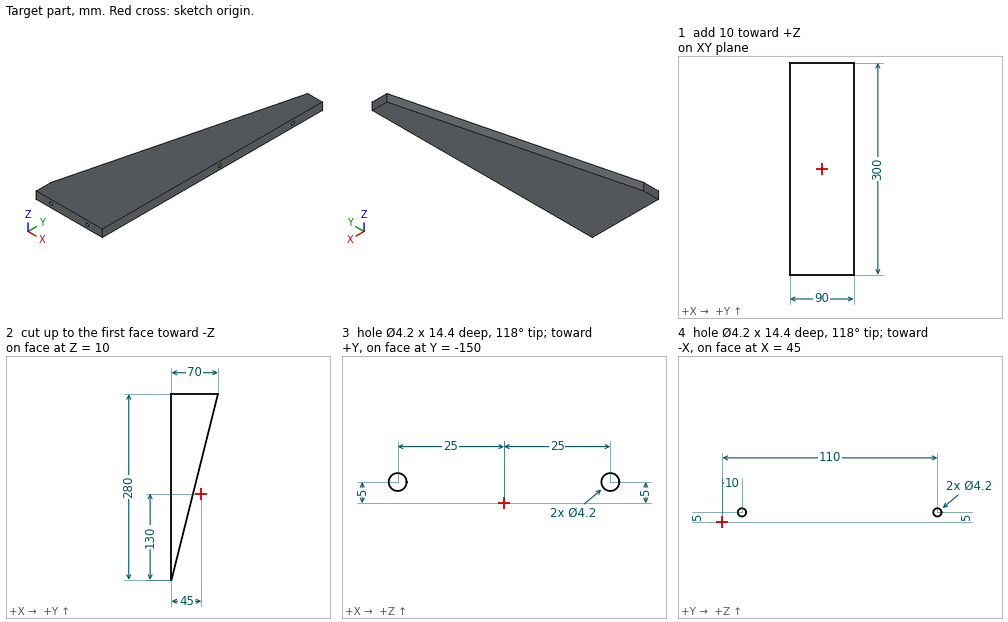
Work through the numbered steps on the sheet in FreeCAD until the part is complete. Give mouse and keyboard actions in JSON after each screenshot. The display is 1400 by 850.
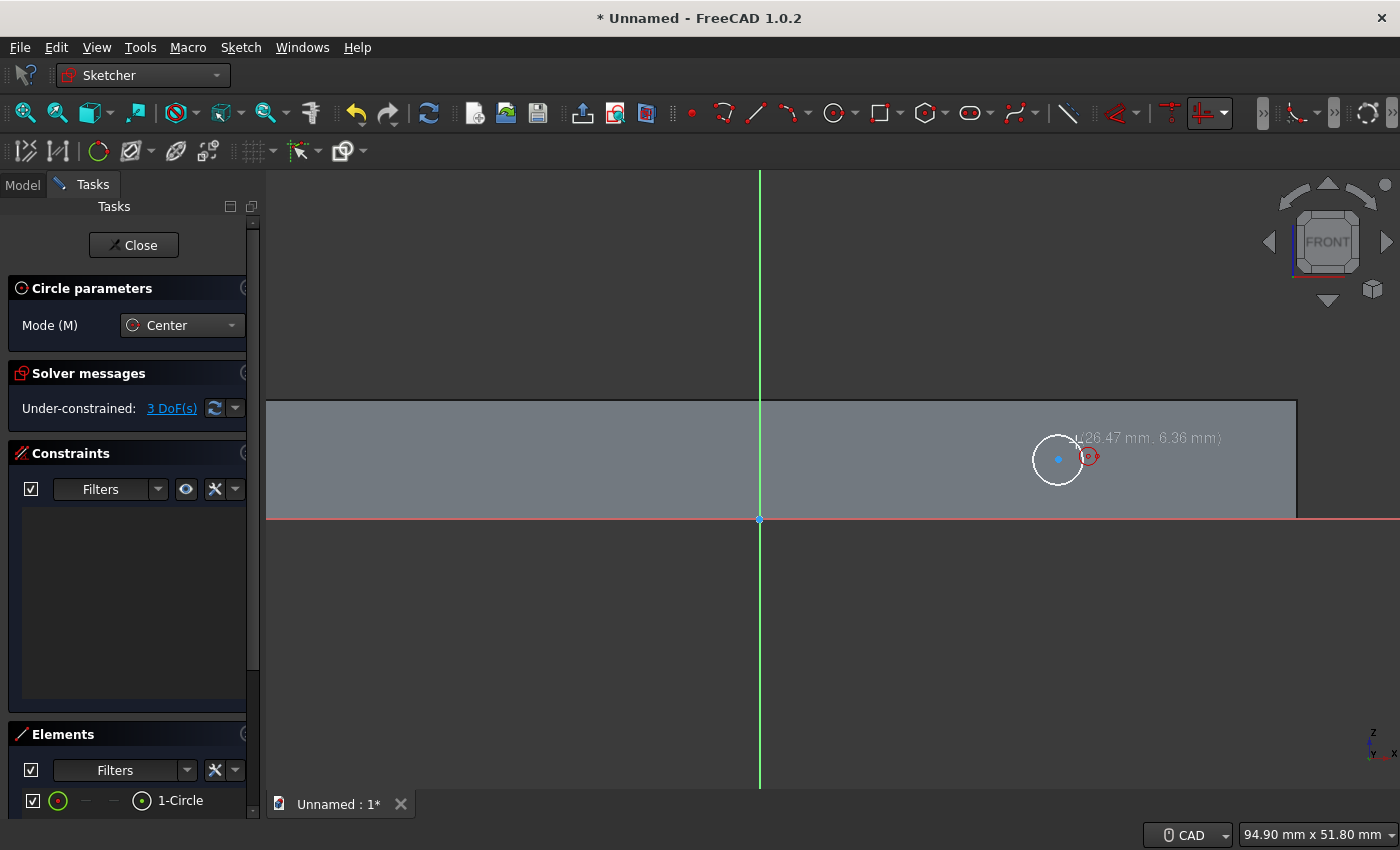
{"action": "left_click", "coordinate": [461, 459]}
{"action": "left_click", "coordinate": [479, 442]}
{"action": "key", "text": "Escape"}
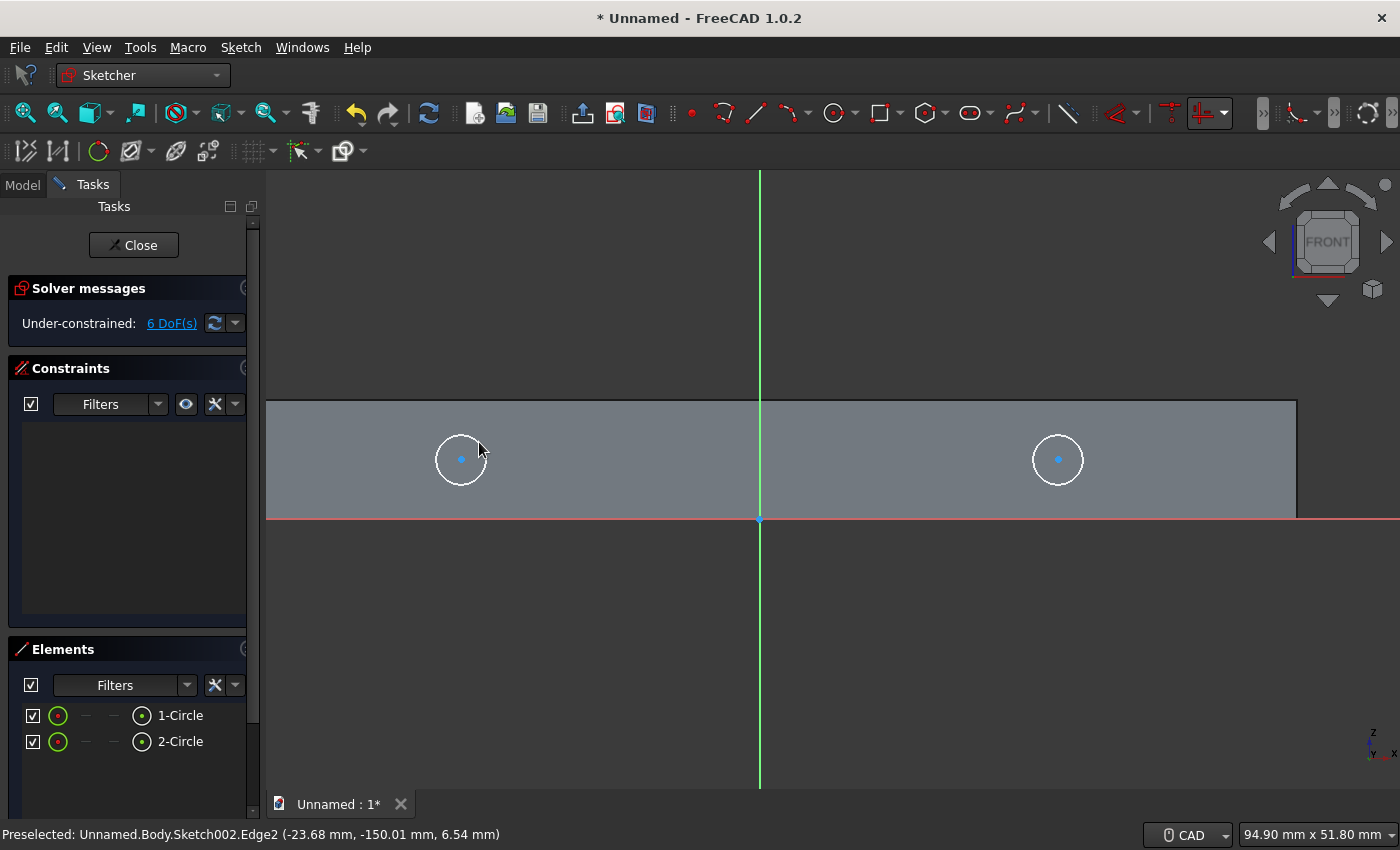
{"action": "left_click", "coordinate": [1075, 442]}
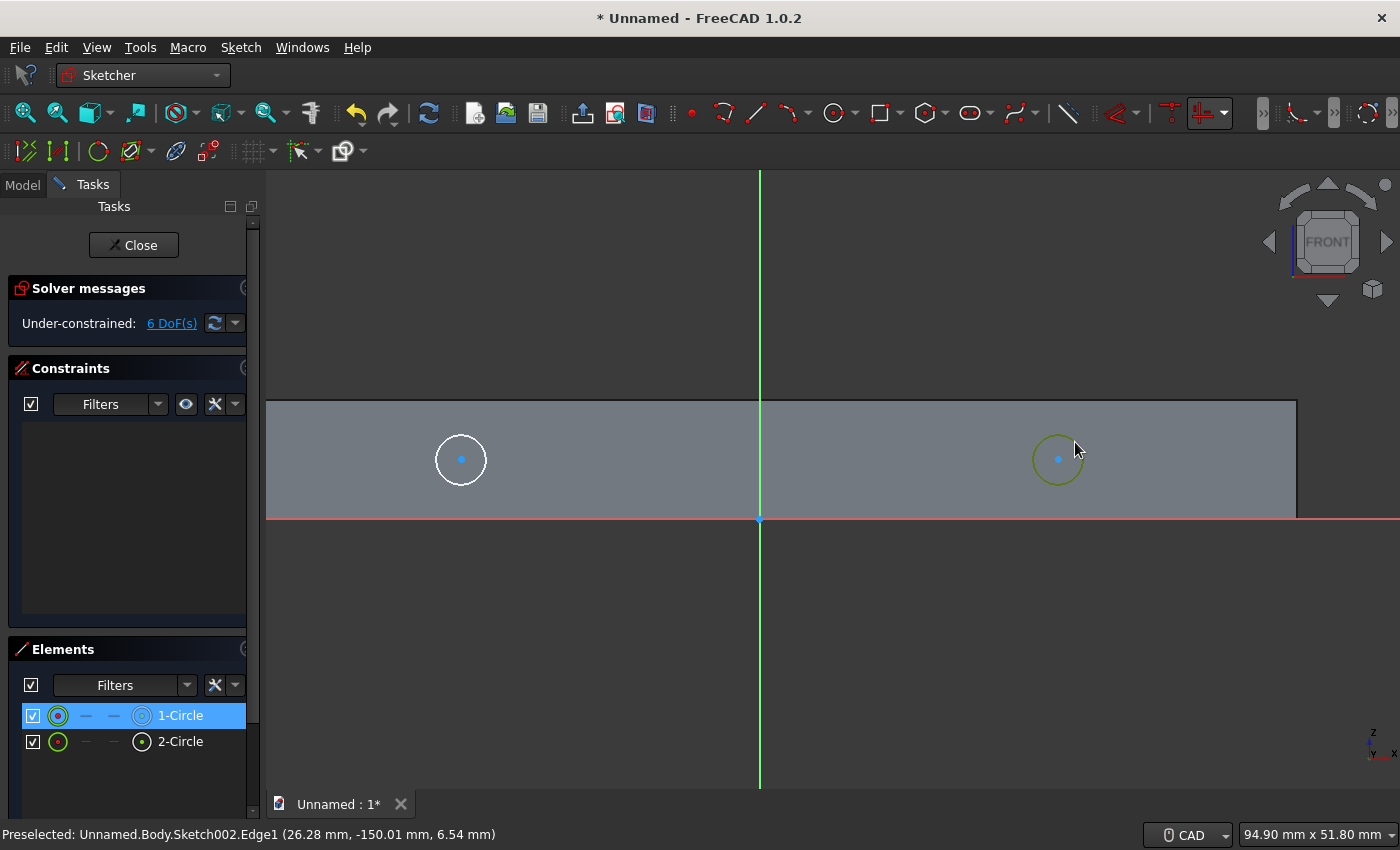
{"action": "left_click", "coordinate": [478, 442]}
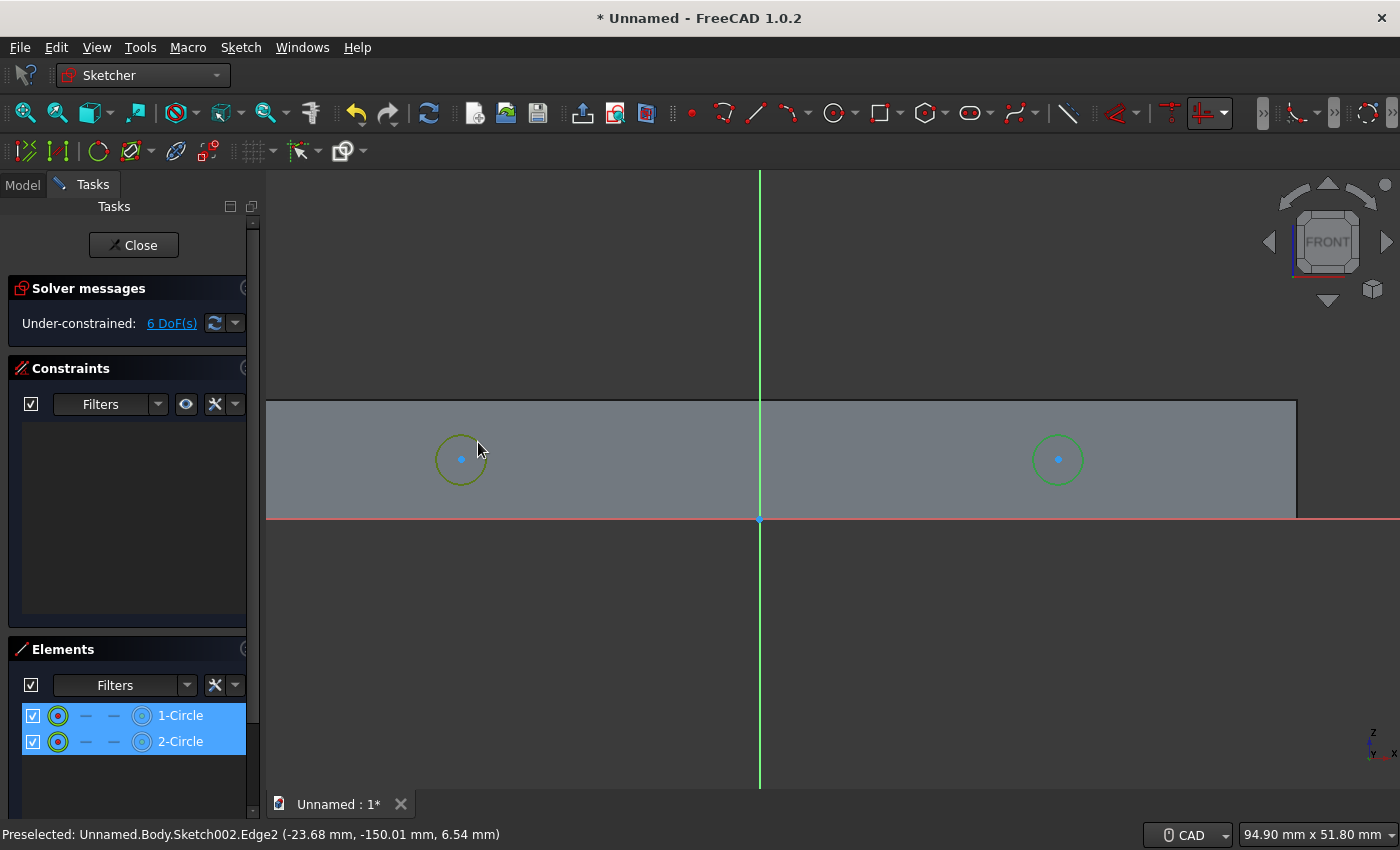
{"action": "key", "text": "e"}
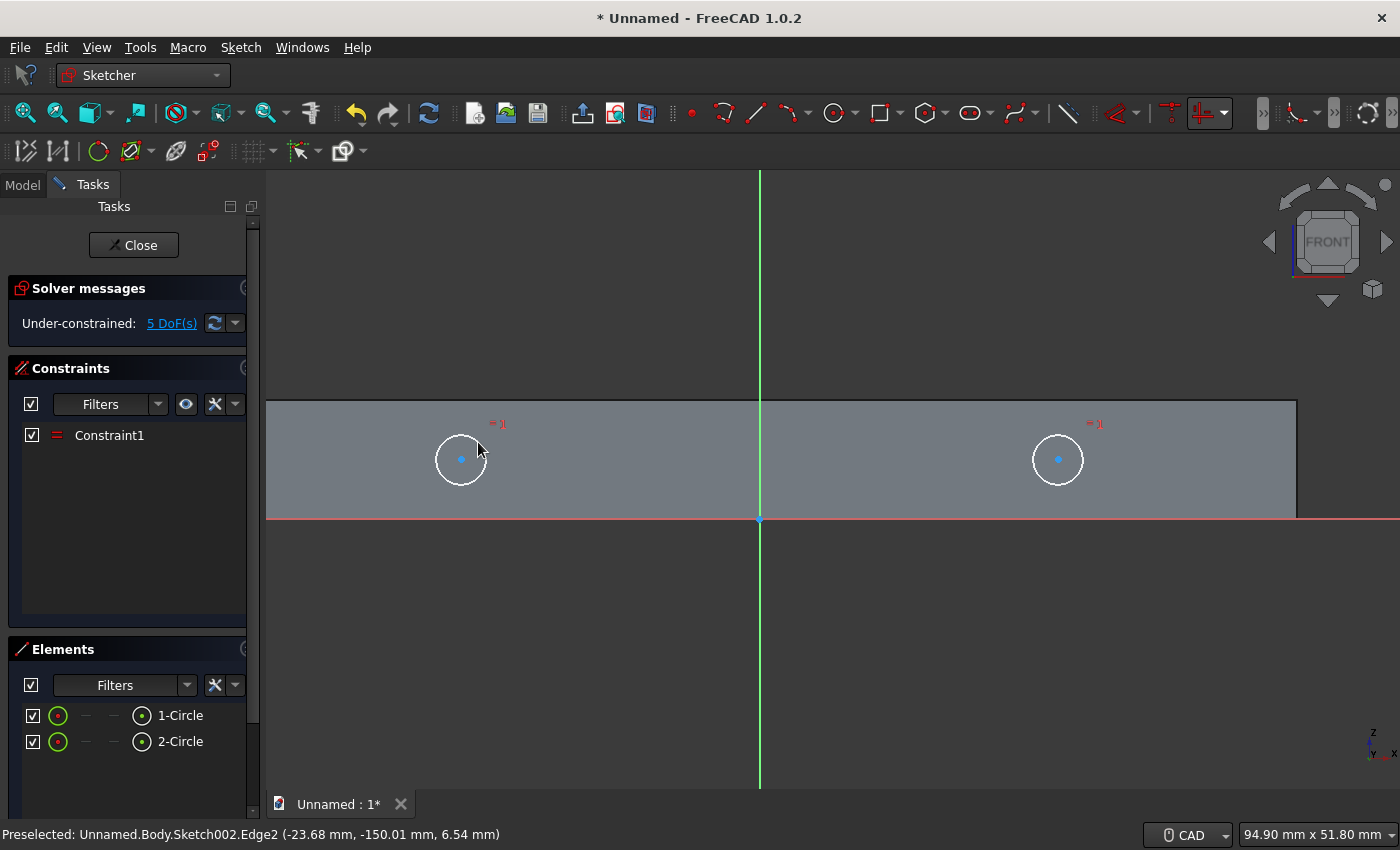
{"action": "left_click", "coordinate": [1116, 114]}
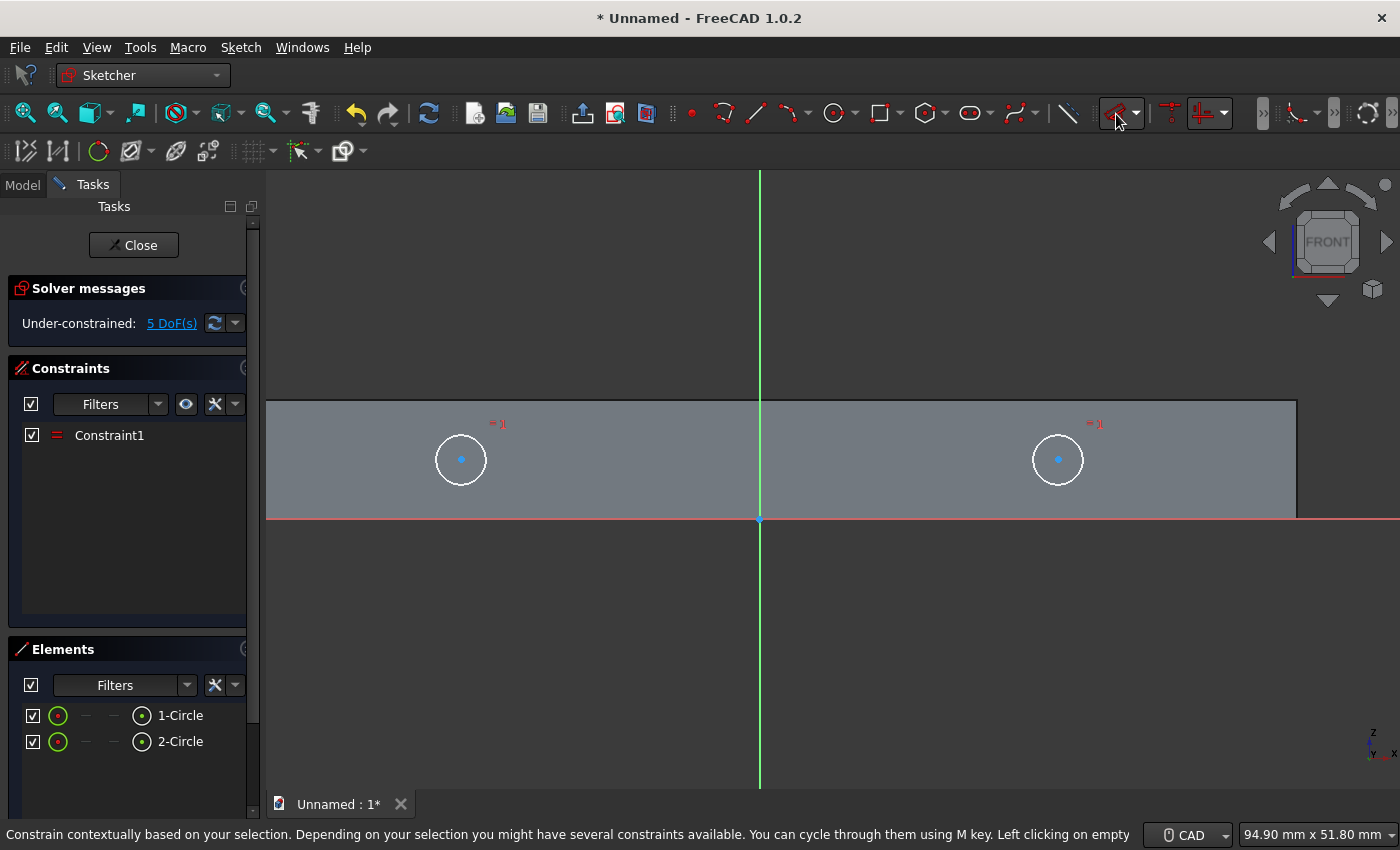
{"action": "left_click", "coordinate": [1075, 442]}
{"action": "left_click", "coordinate": [1097, 419]}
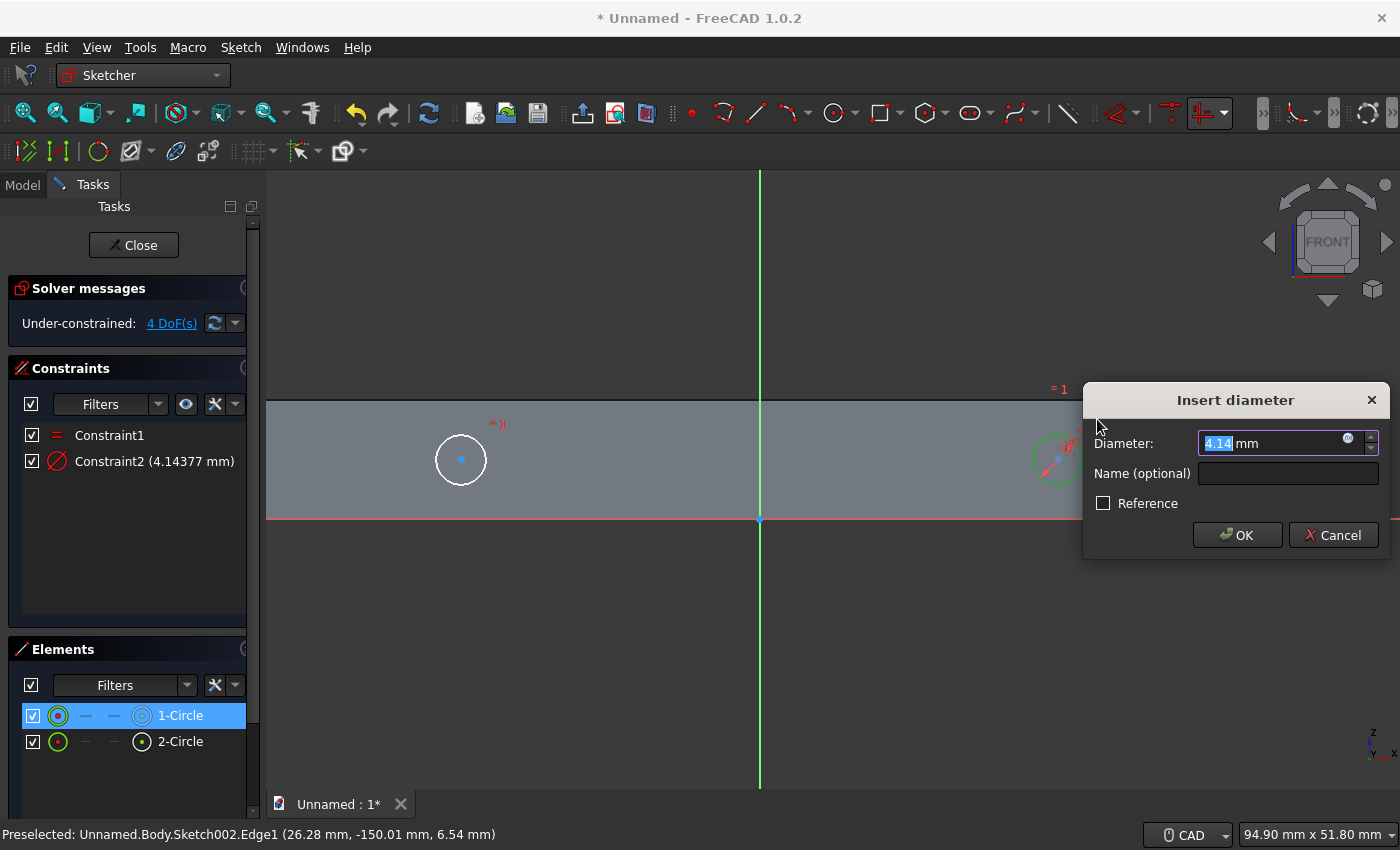
{"action": "type", "text": "4.2"}
{"action": "key", "text": "Return"}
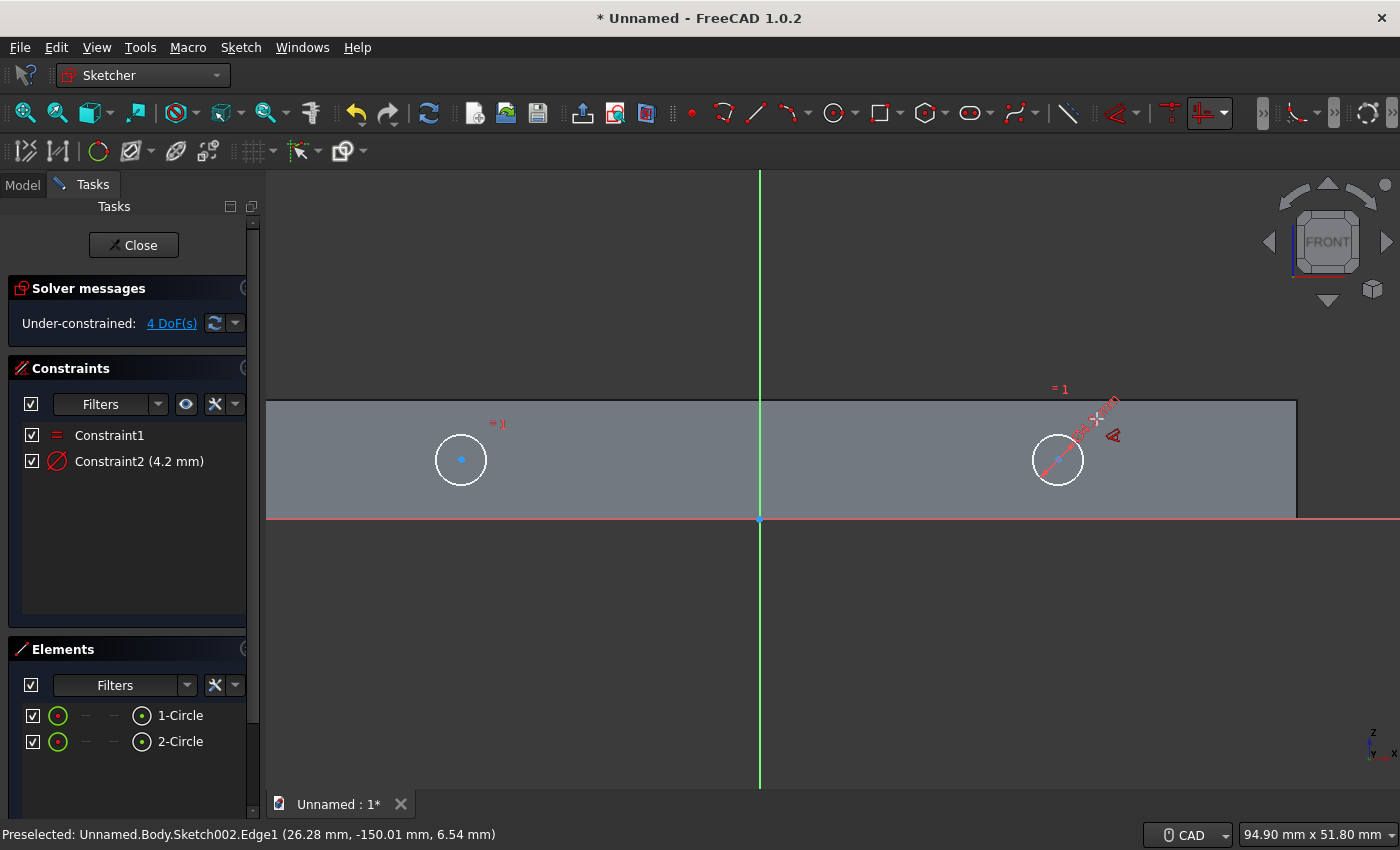
{"action": "left_click", "coordinate": [1058, 460]}
{"action": "left_click", "coordinate": [1092, 490]}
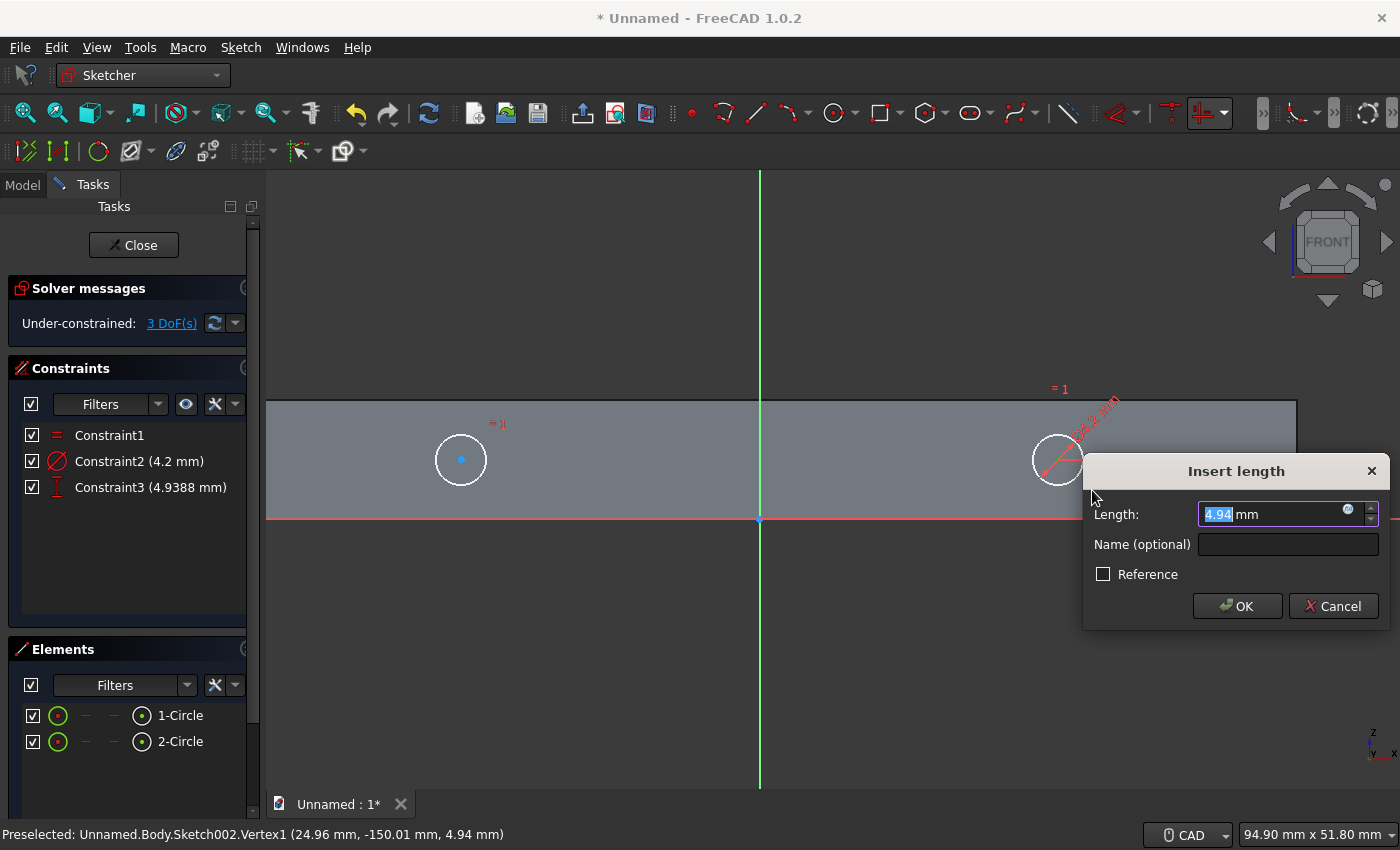
{"action": "type", "text": "5"}
{"action": "key", "text": "Return"}